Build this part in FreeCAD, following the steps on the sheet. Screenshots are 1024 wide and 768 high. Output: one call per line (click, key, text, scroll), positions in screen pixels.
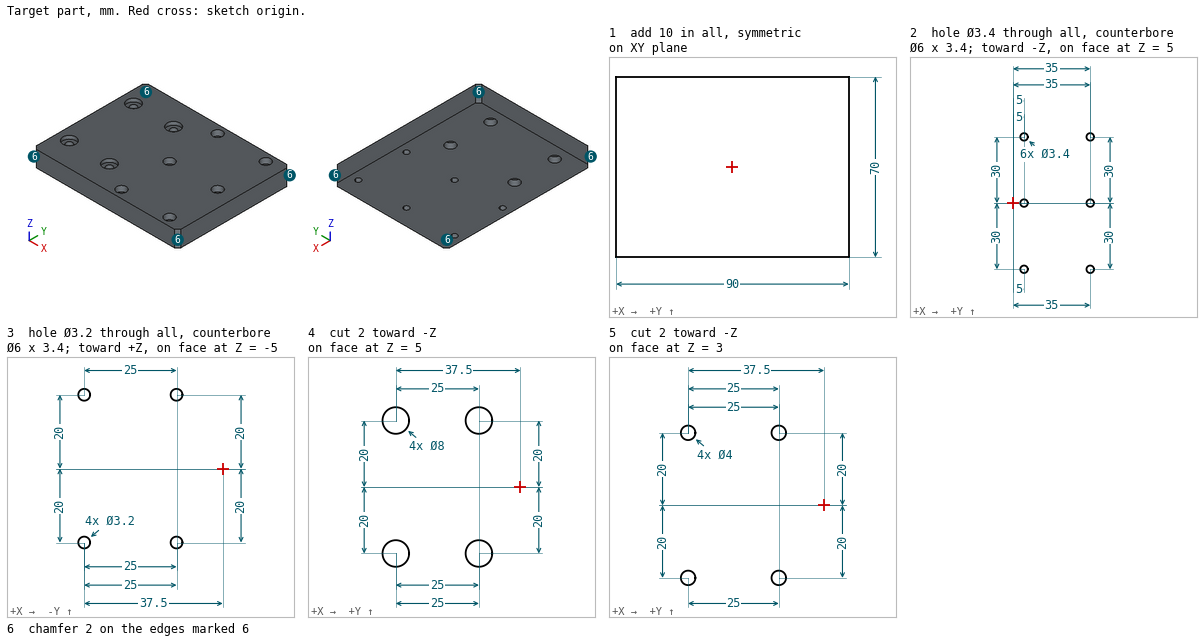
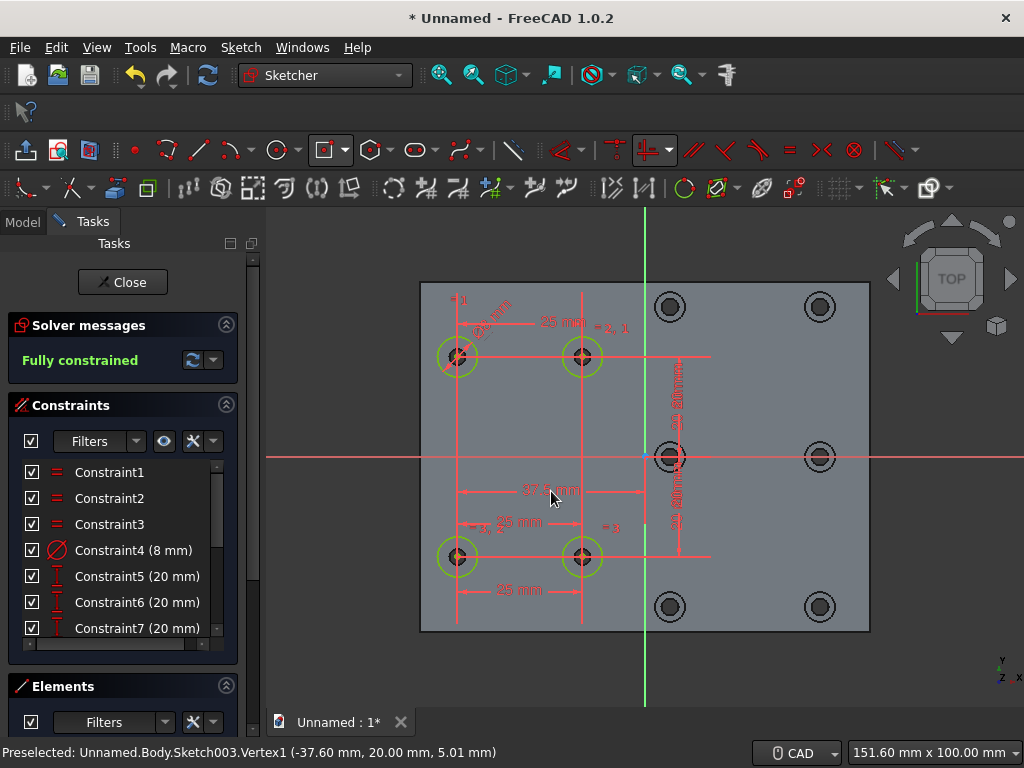
click(123, 282)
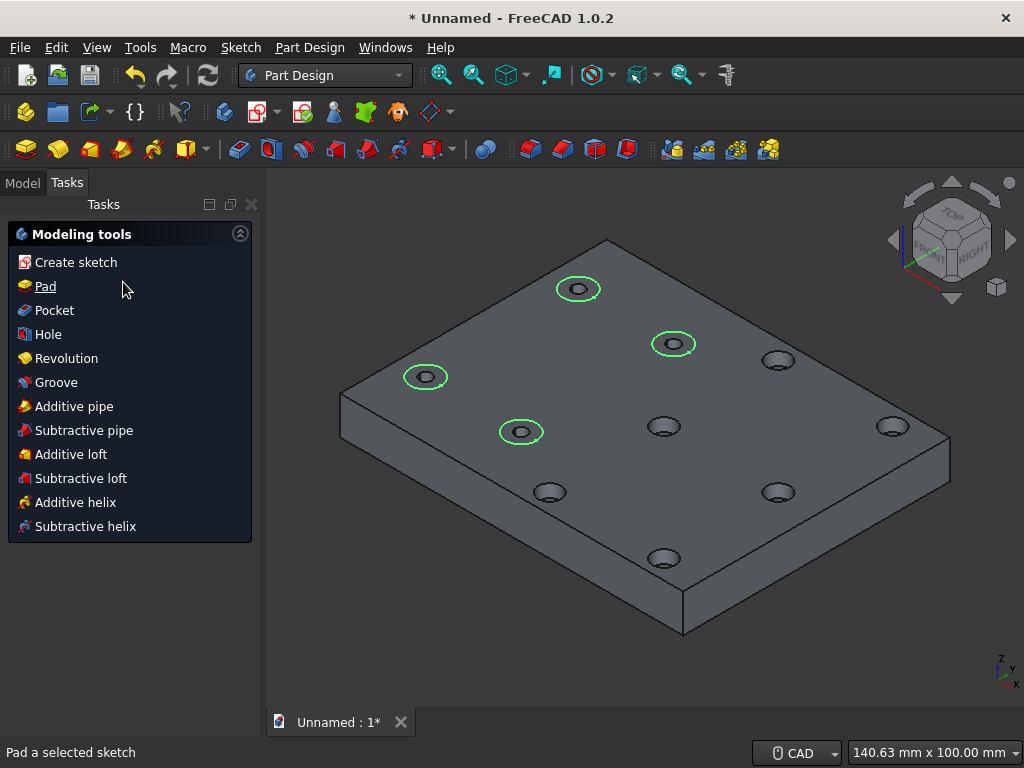
click(240, 150)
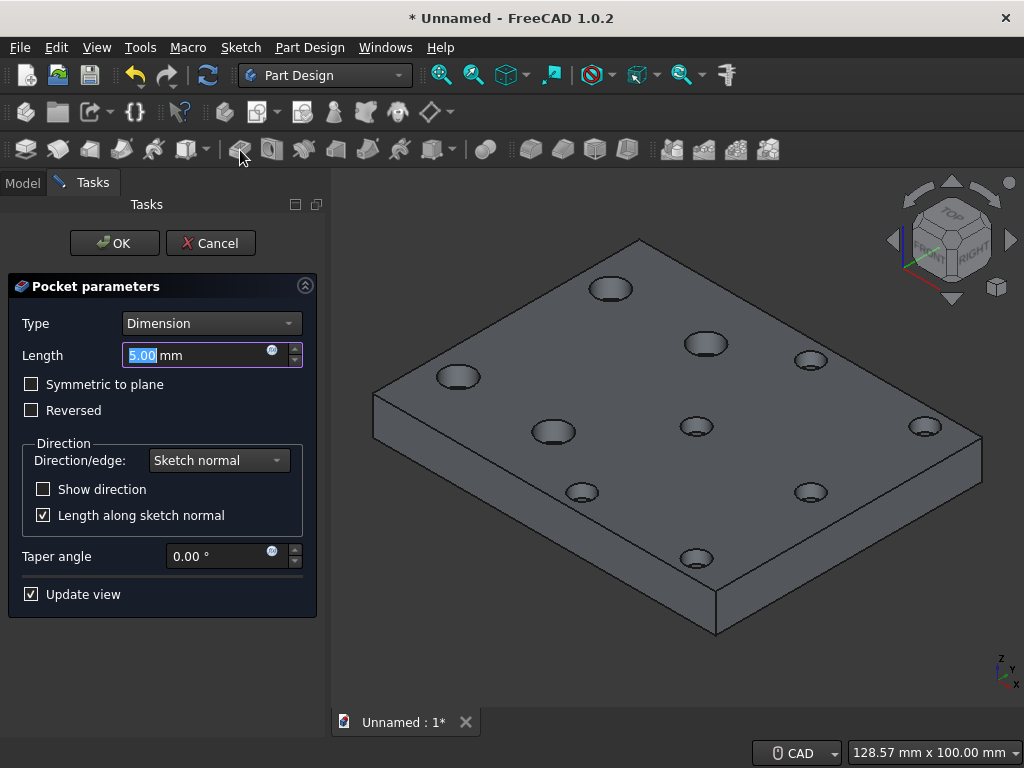
text(2)
key(Tab)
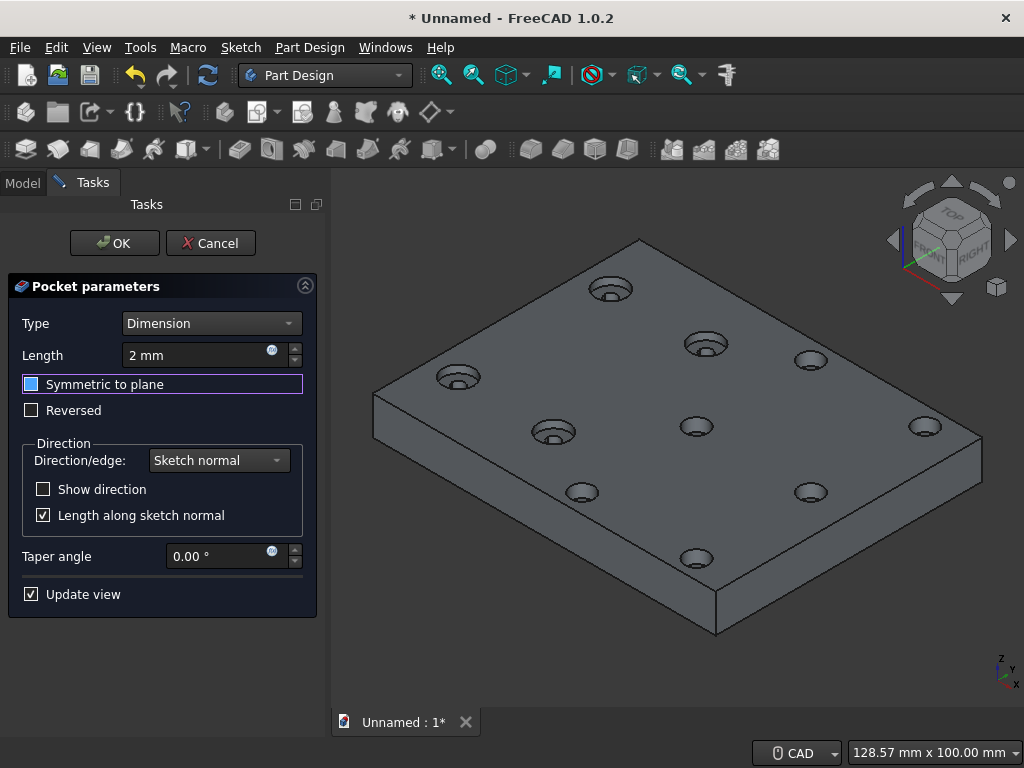
click(115, 243)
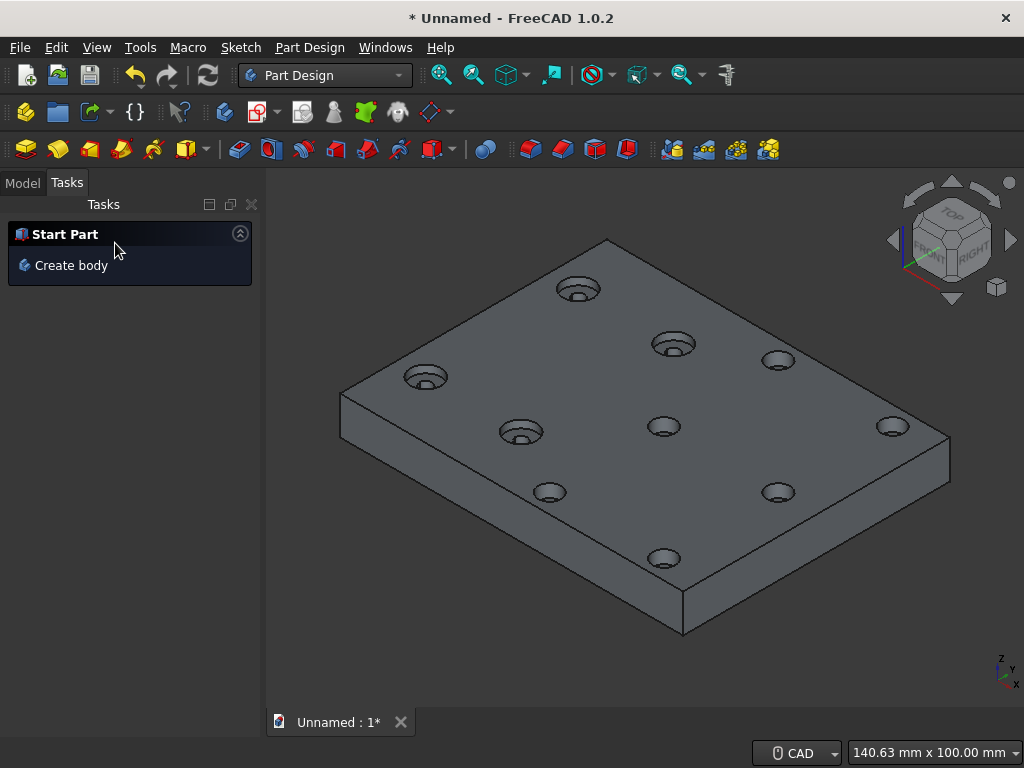
scroll(517, 432, up, 5)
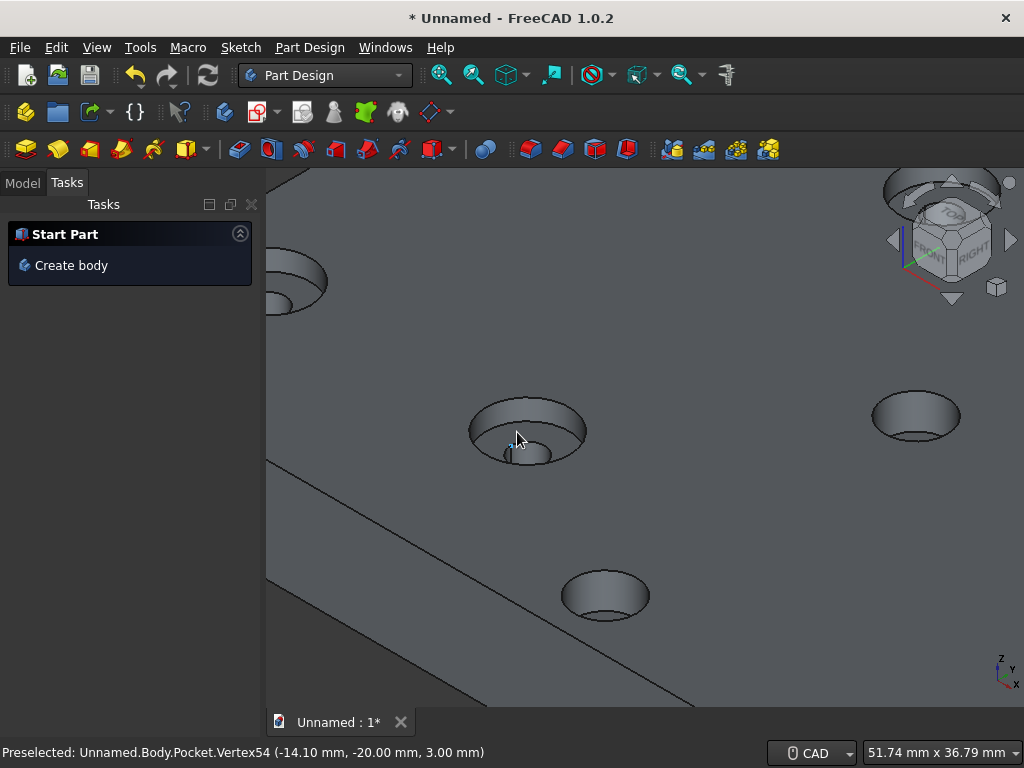
click(442, 76)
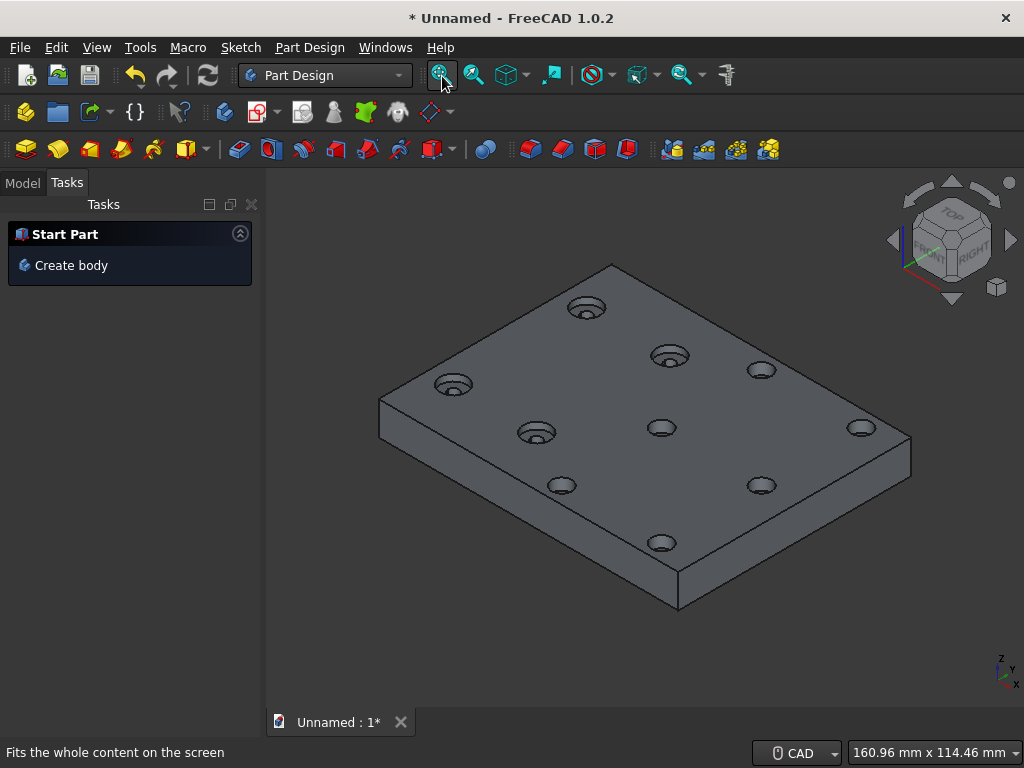
key(2)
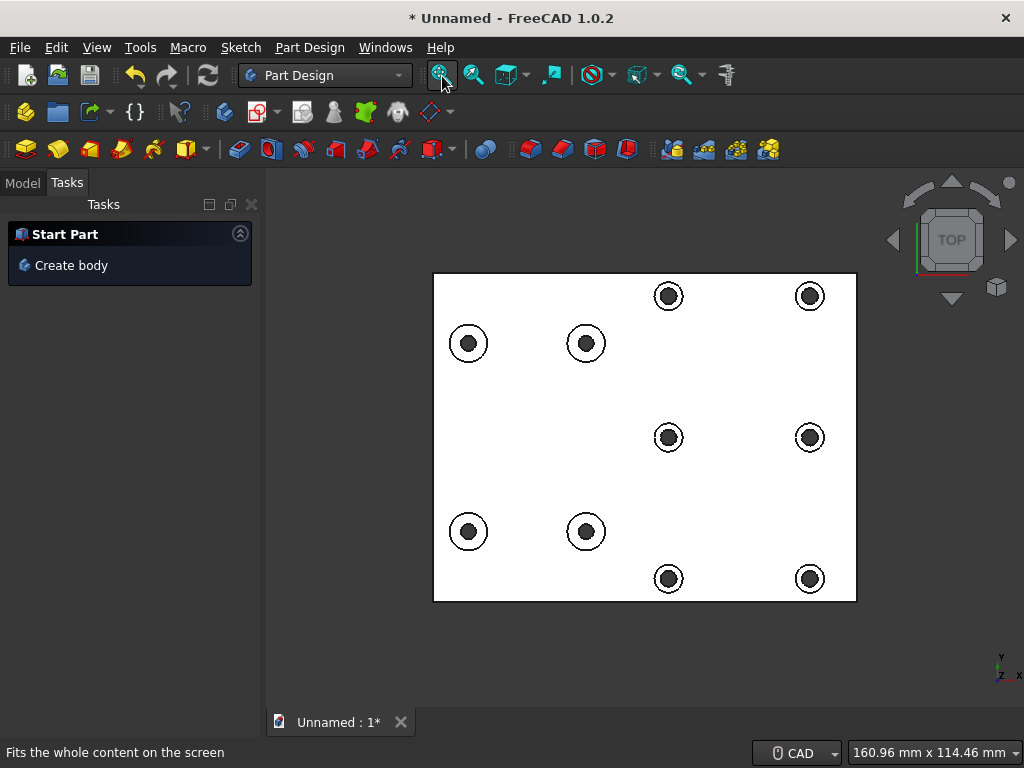
scroll(575, 525, up, 5)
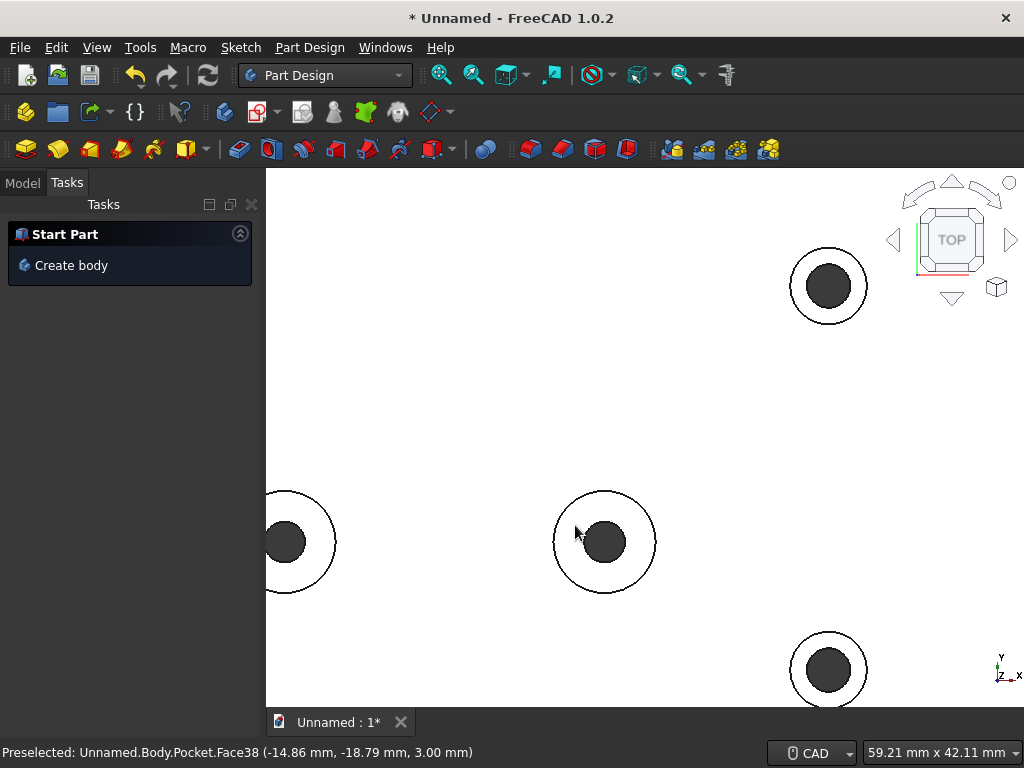
click(575, 526)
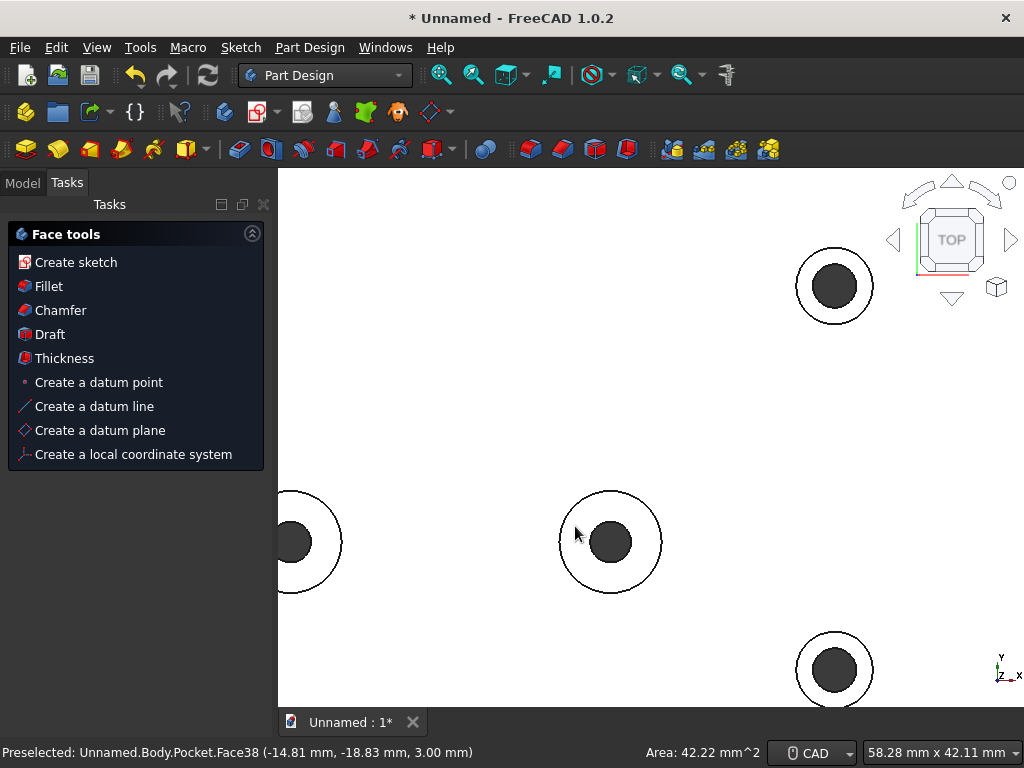
click(258, 112)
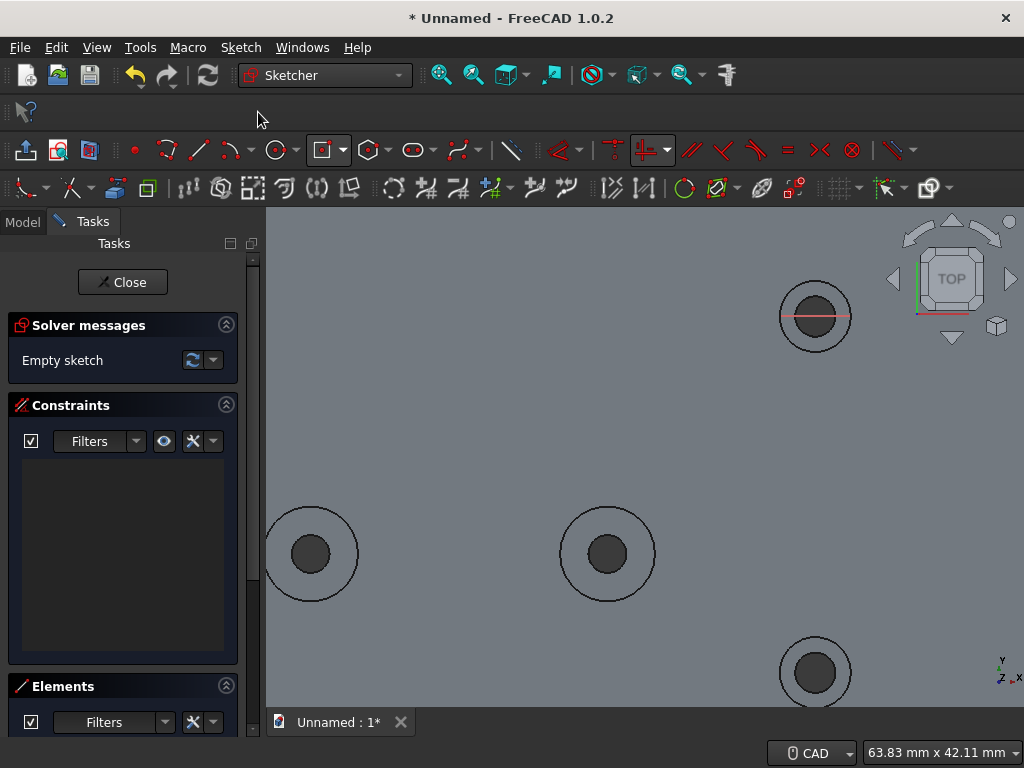
scroll(644, 628, down, 3)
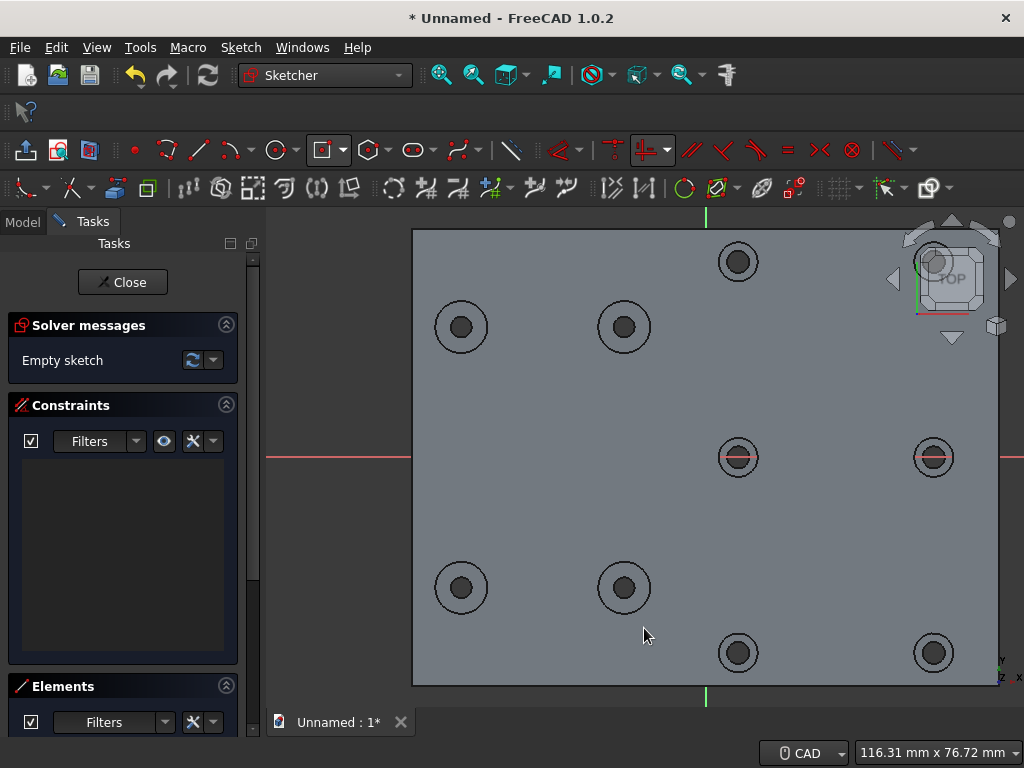
click(276, 150)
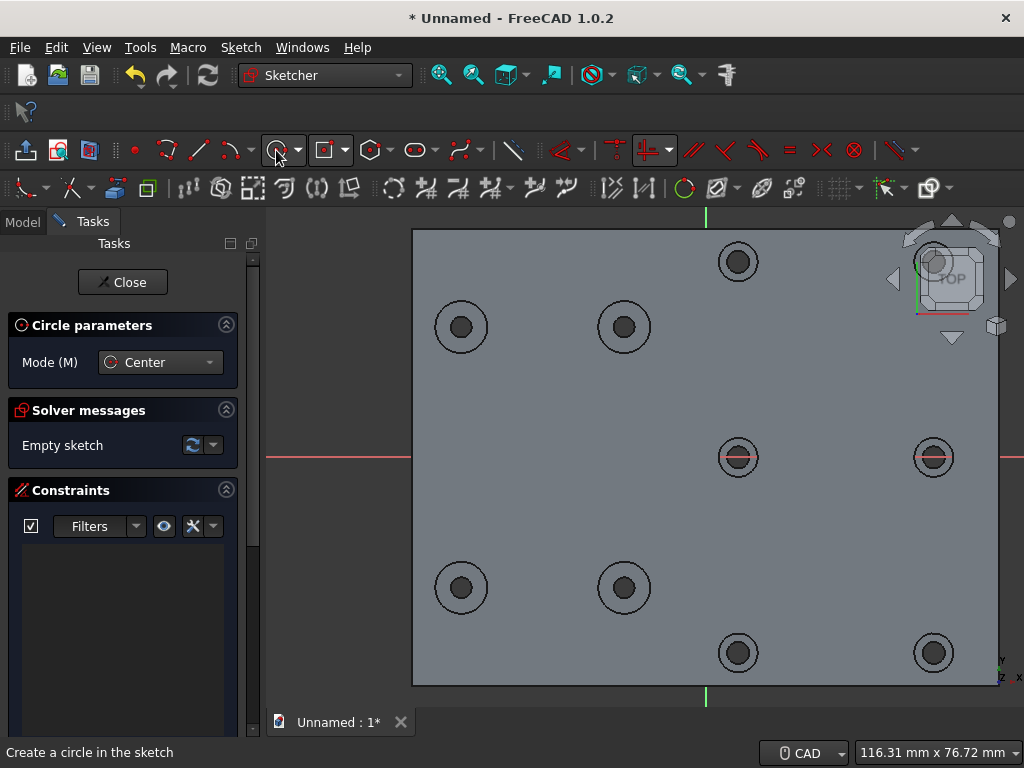
scroll(461, 327, up, 3)